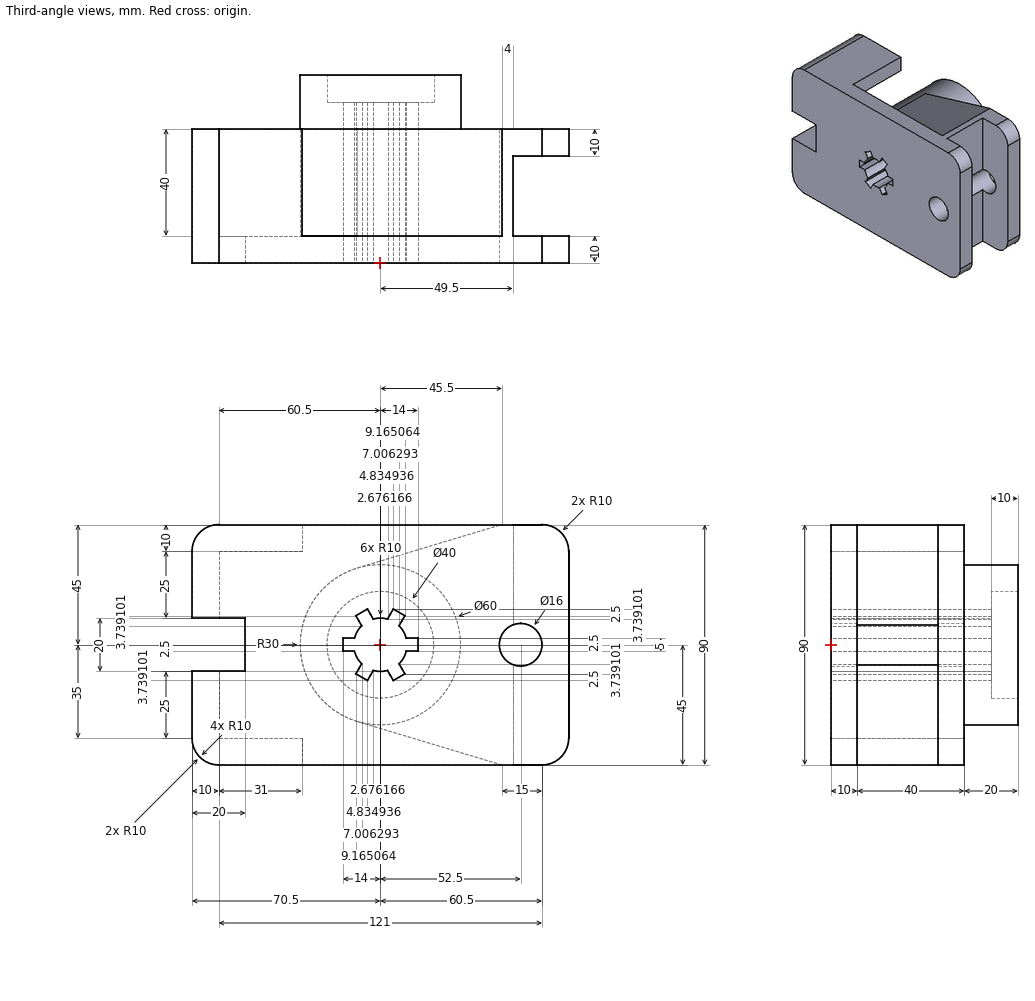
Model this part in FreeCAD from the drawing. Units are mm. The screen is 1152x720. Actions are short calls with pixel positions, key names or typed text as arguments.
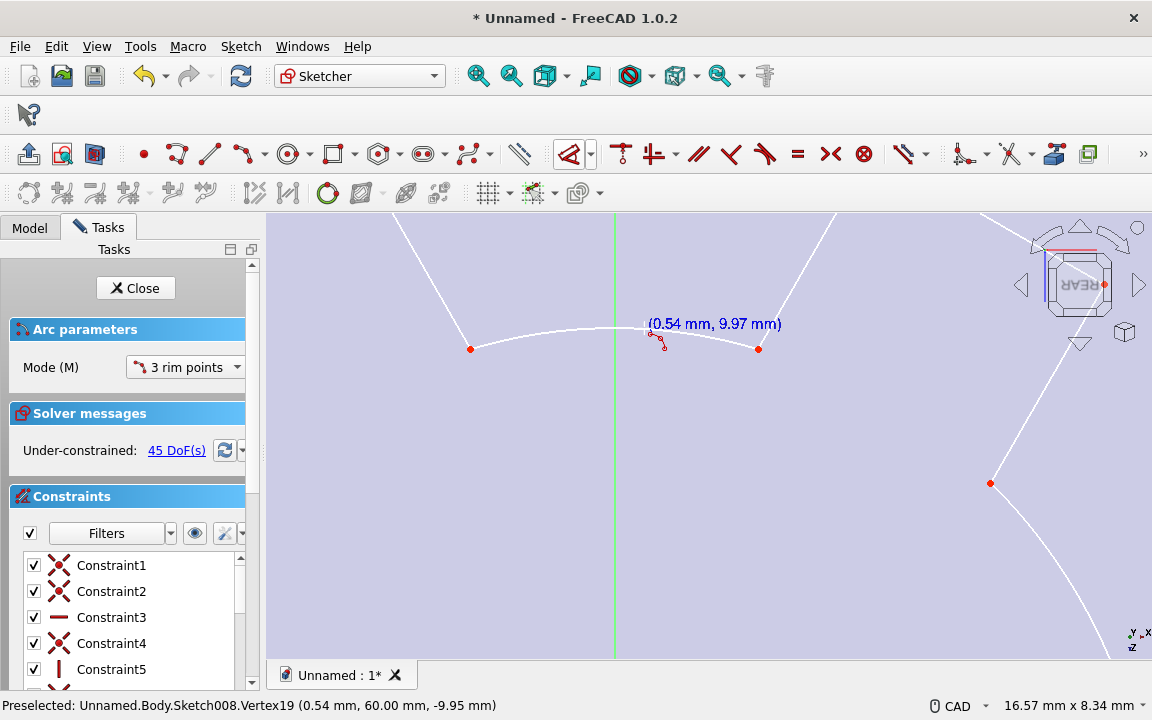
scroll(647, 328, down, 8)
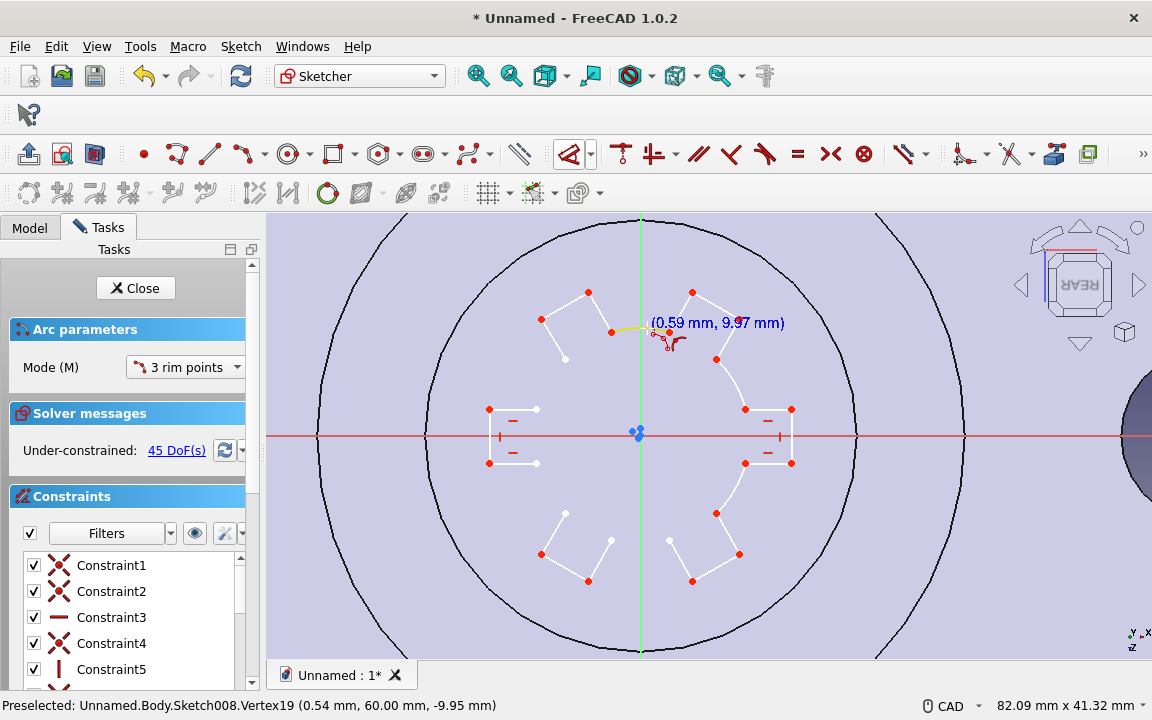
click(566, 360)
click(537, 410)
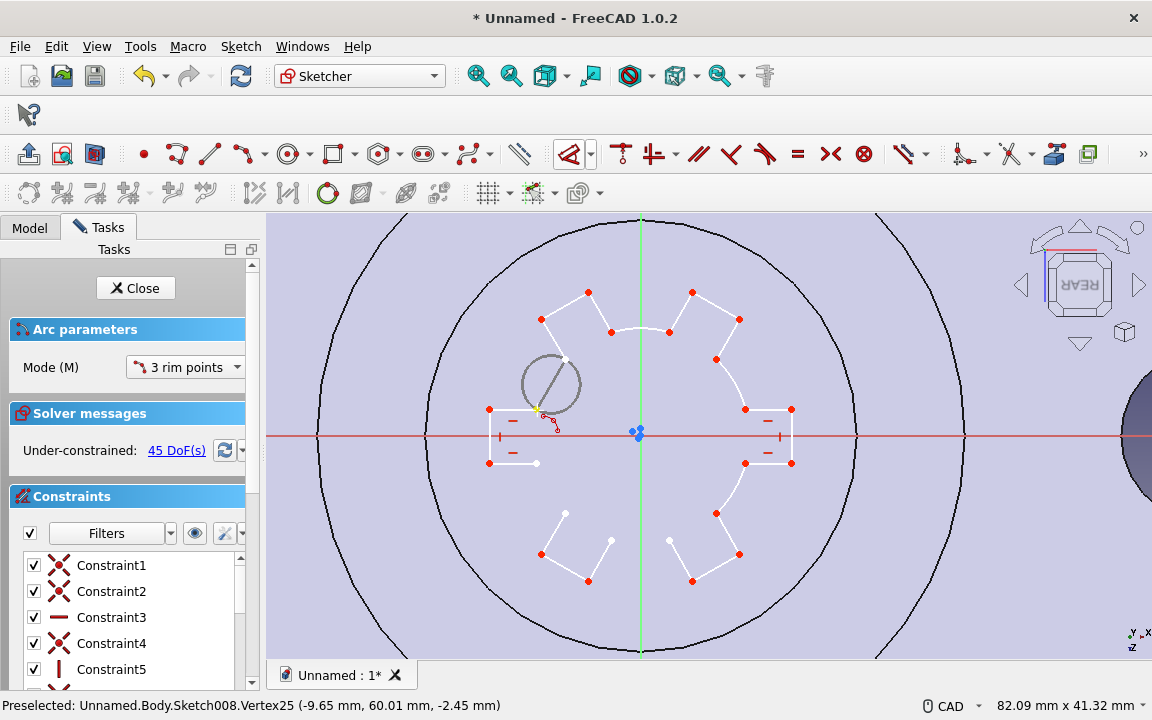
scroll(547, 382, up, 7)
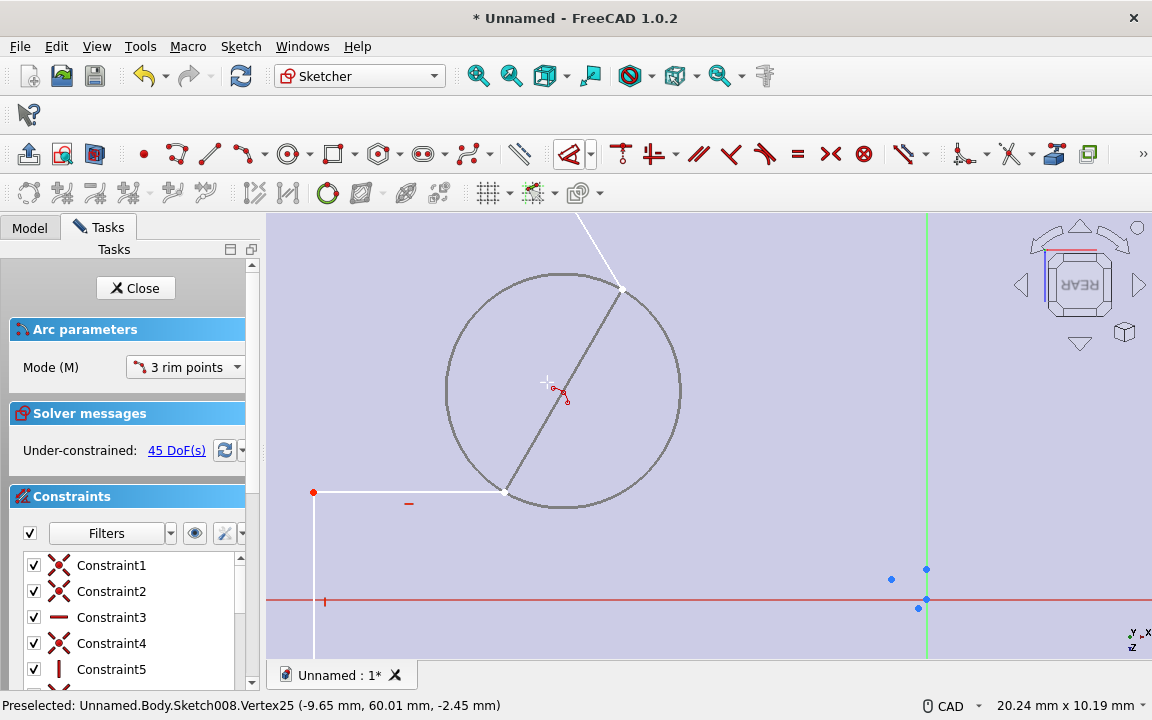
click(548, 381)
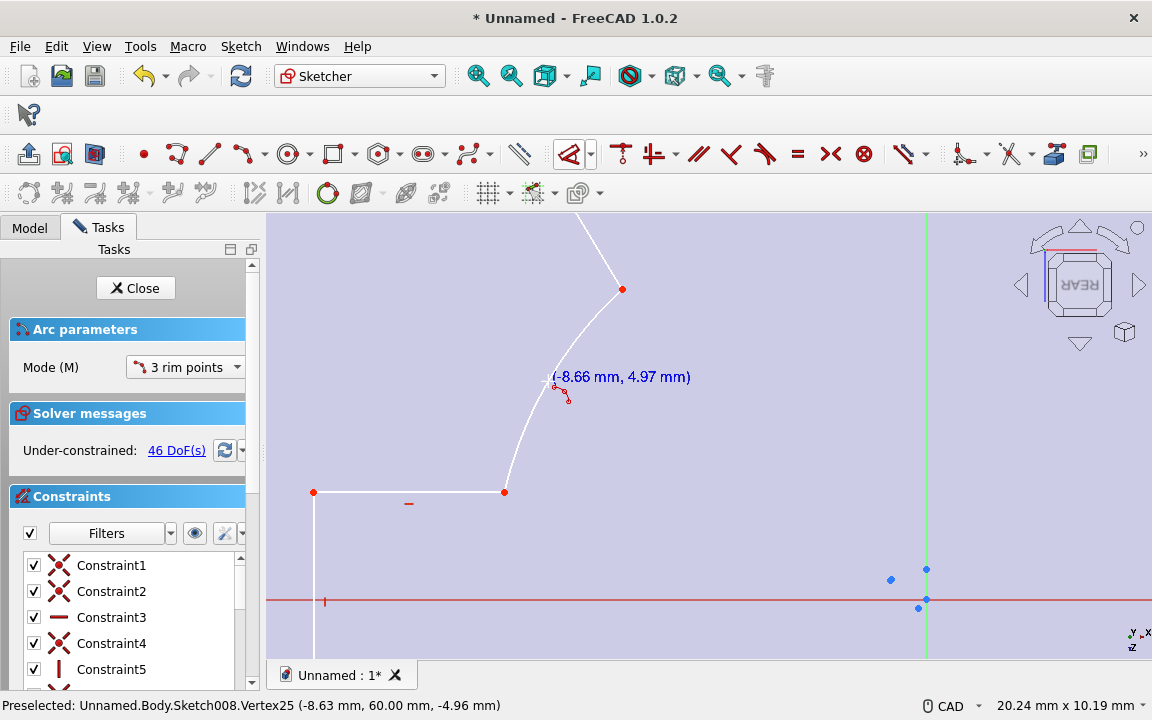
scroll(547, 382, down, 7)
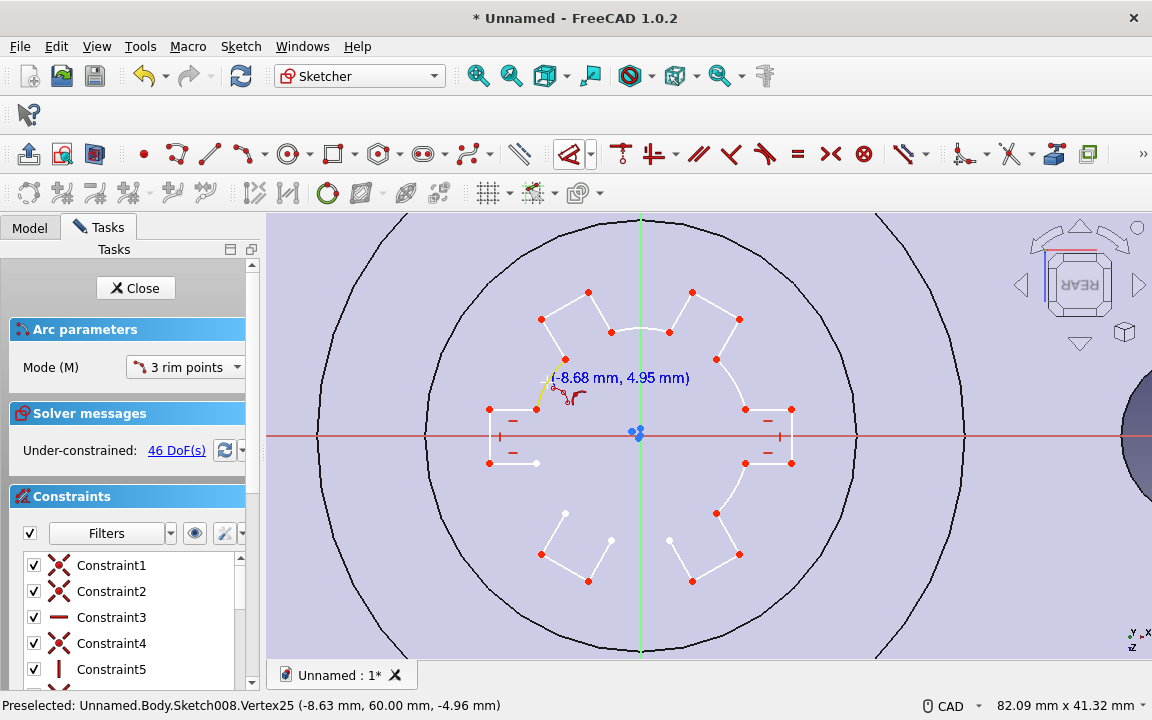
click(537, 464)
click(566, 514)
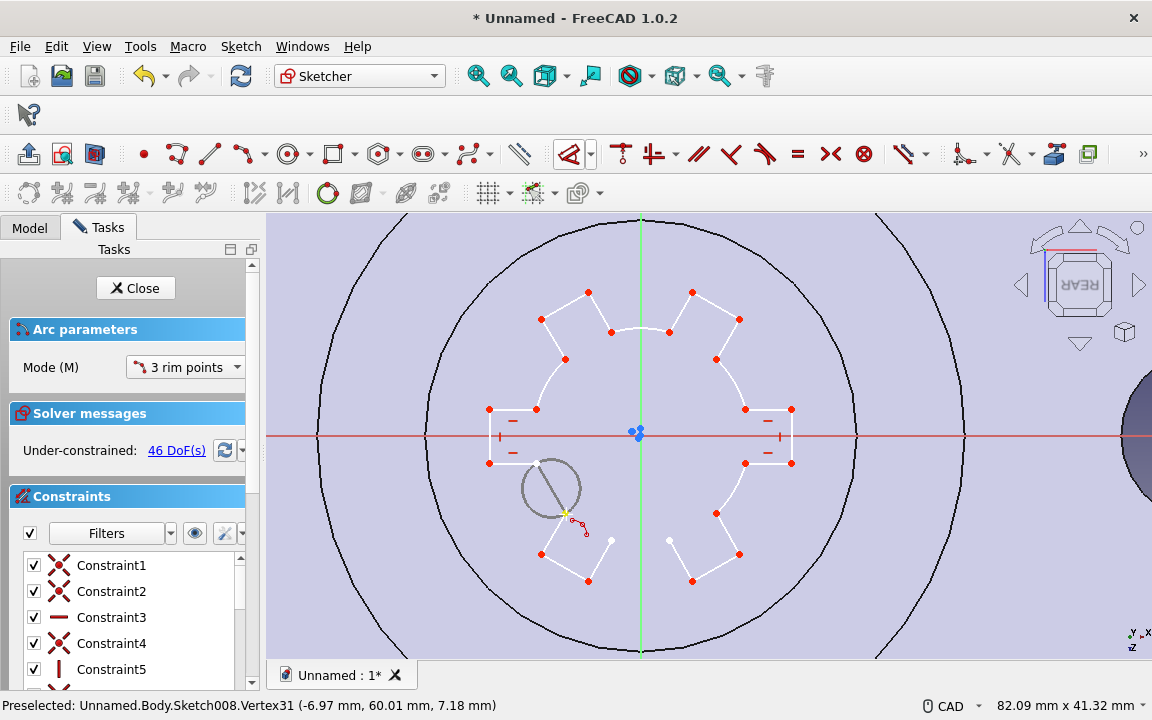
scroll(547, 490, up, 7)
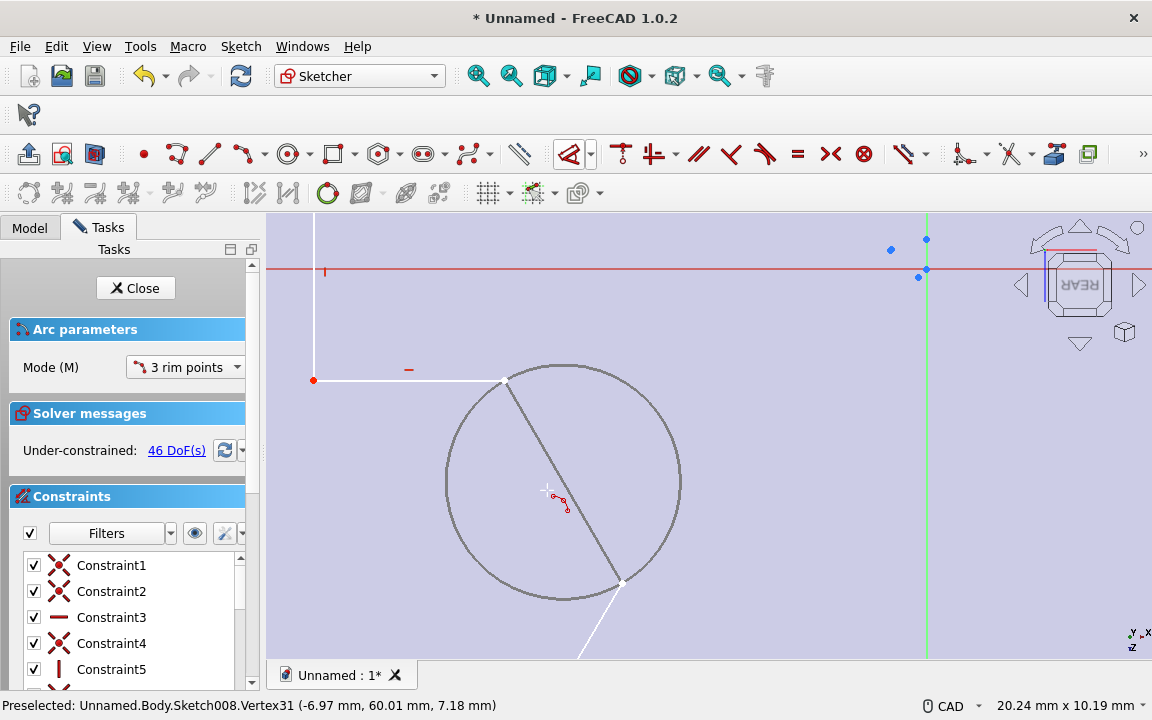
click(548, 488)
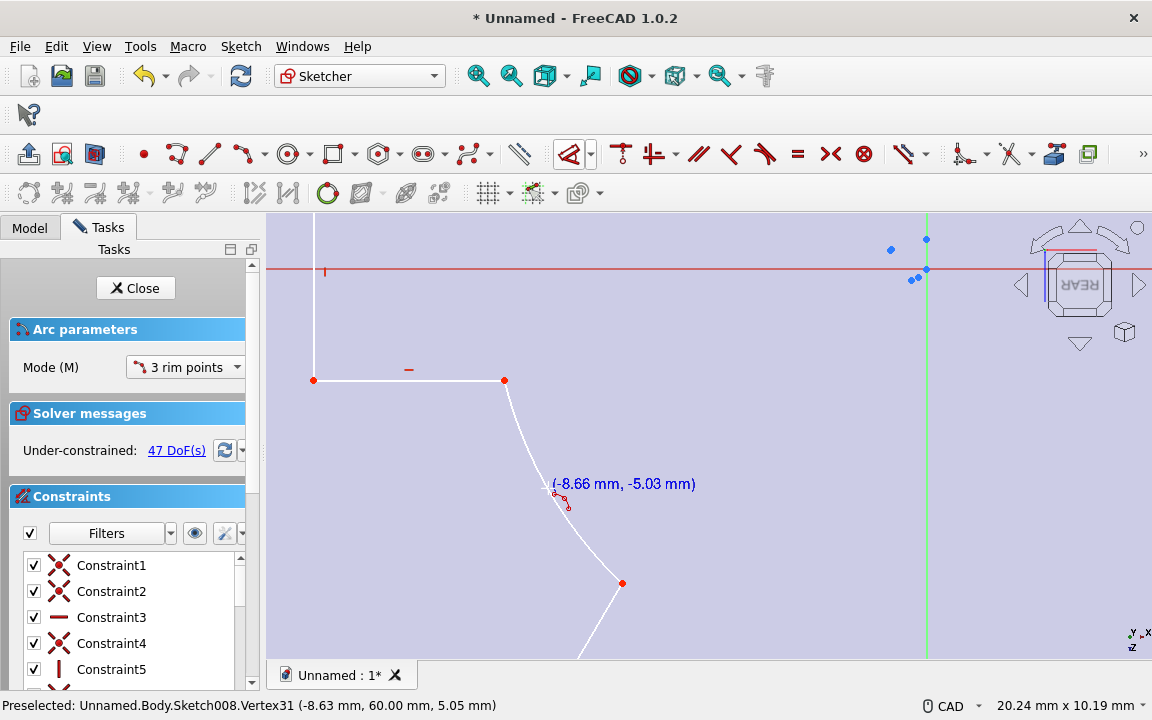
scroll(547, 491, down, 7)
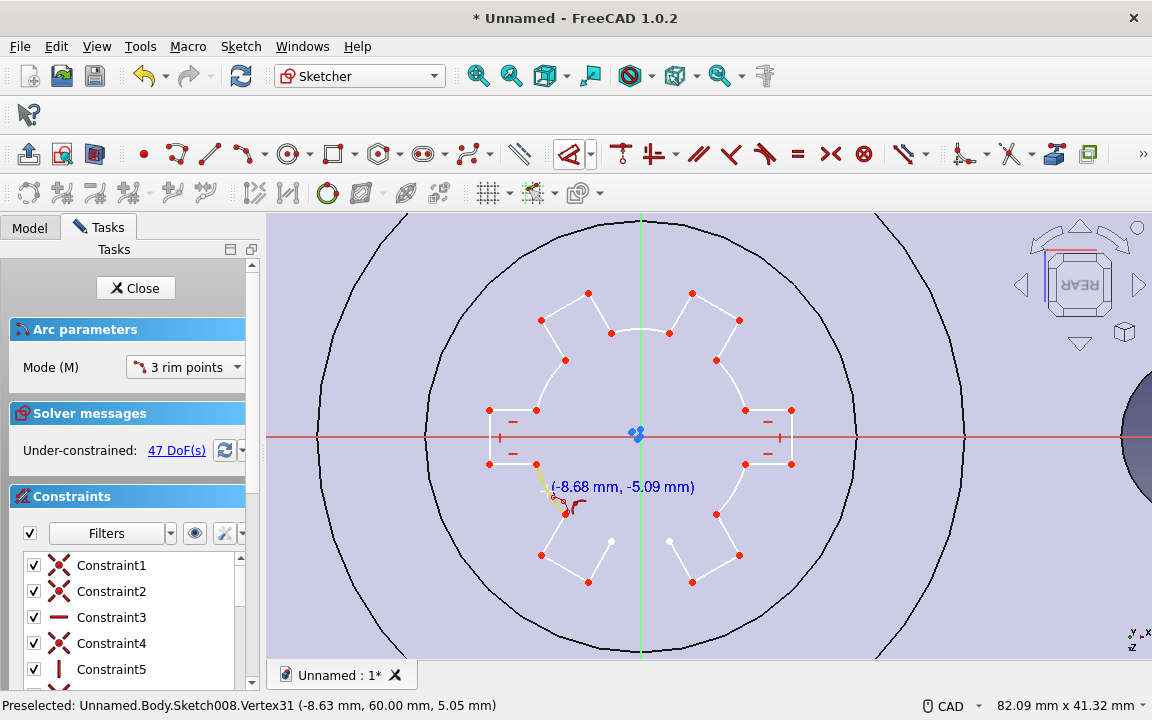
click(612, 541)
click(670, 541)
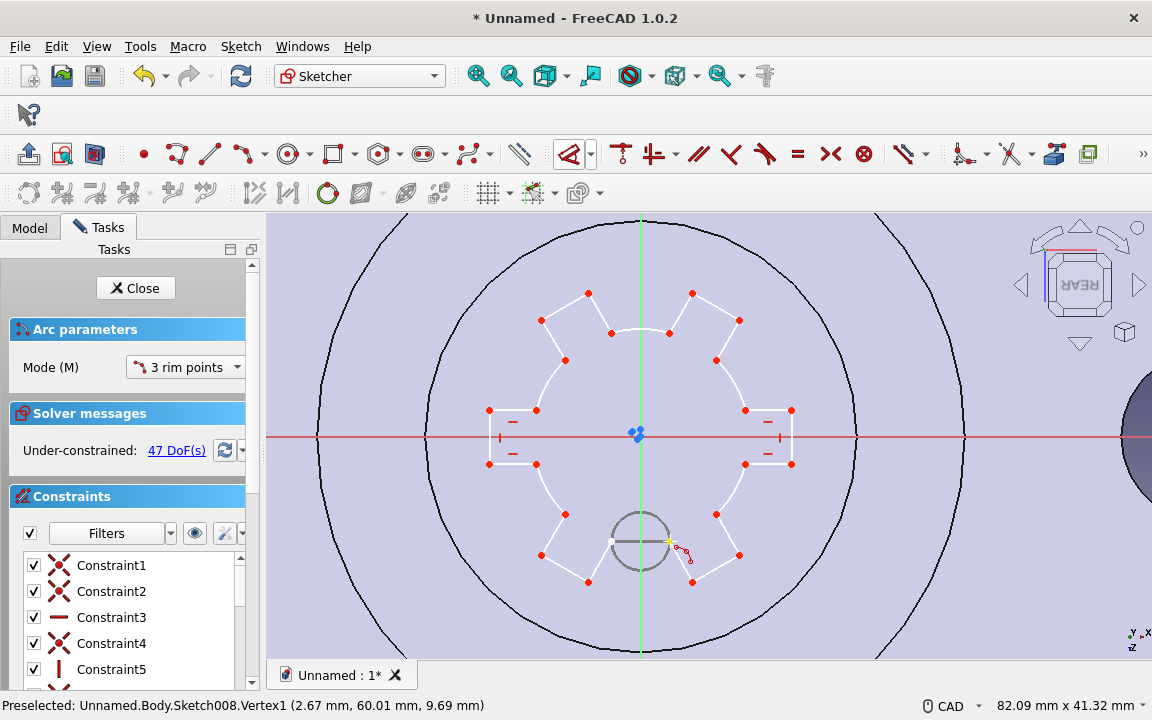
scroll(635, 545, up, 8)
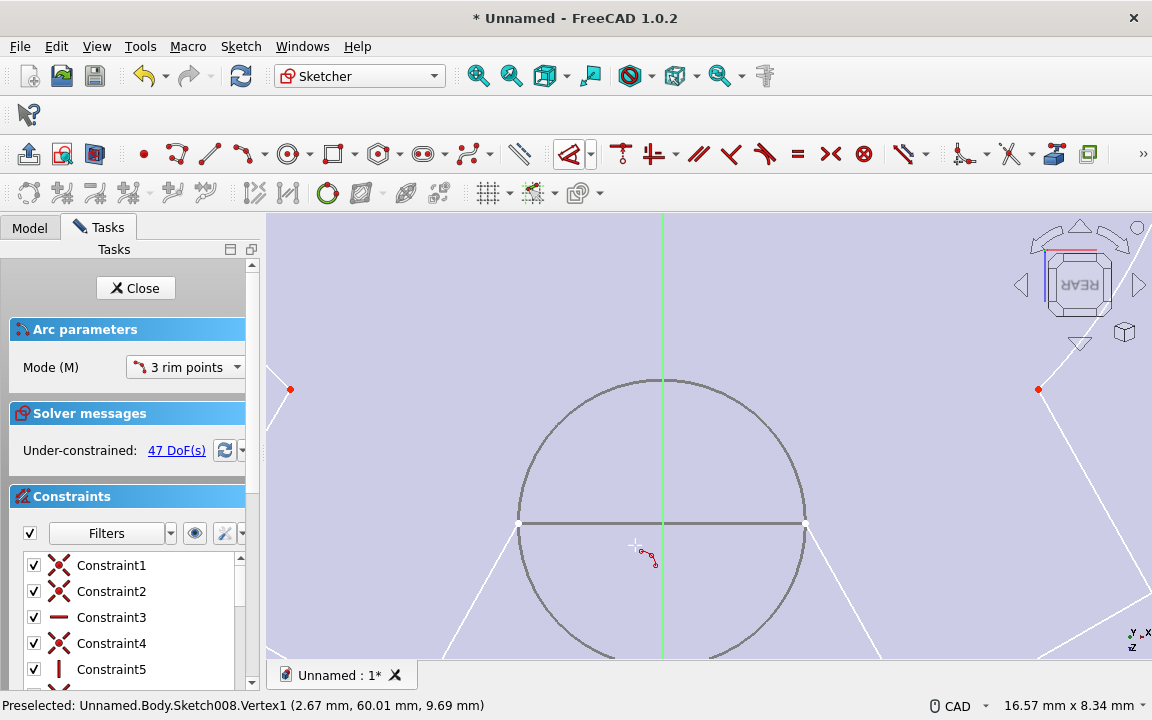
click(634, 540)
key(Escape)